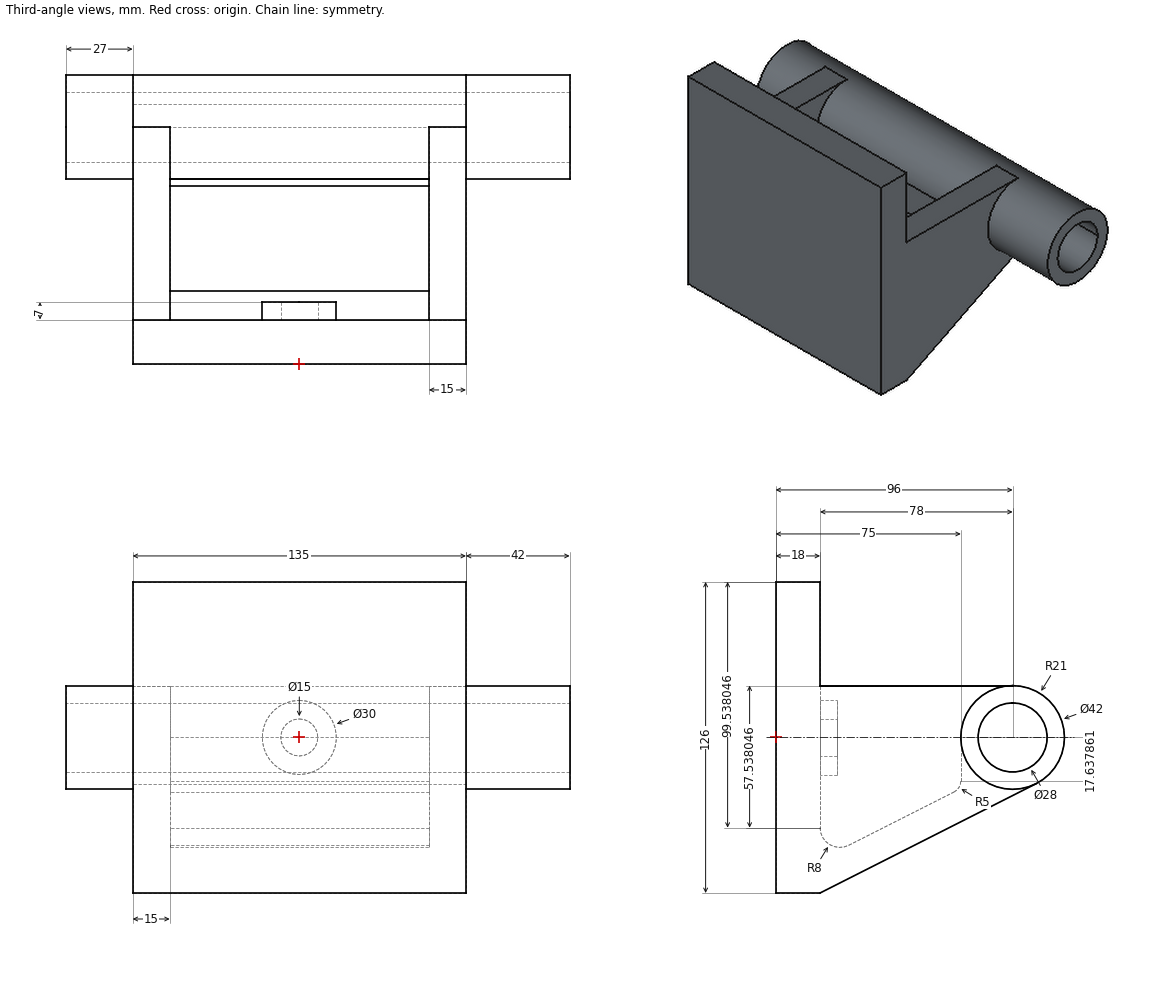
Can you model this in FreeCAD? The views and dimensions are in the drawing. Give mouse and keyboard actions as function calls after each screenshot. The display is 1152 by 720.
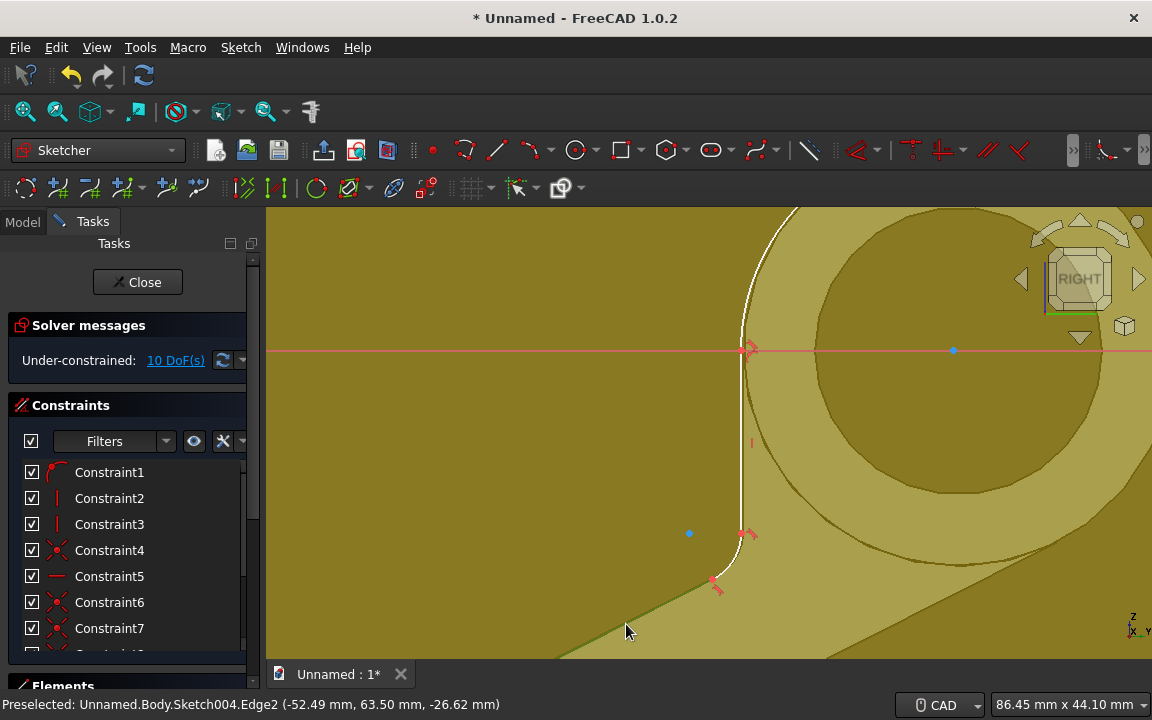
scroll(782, 405, down, 4)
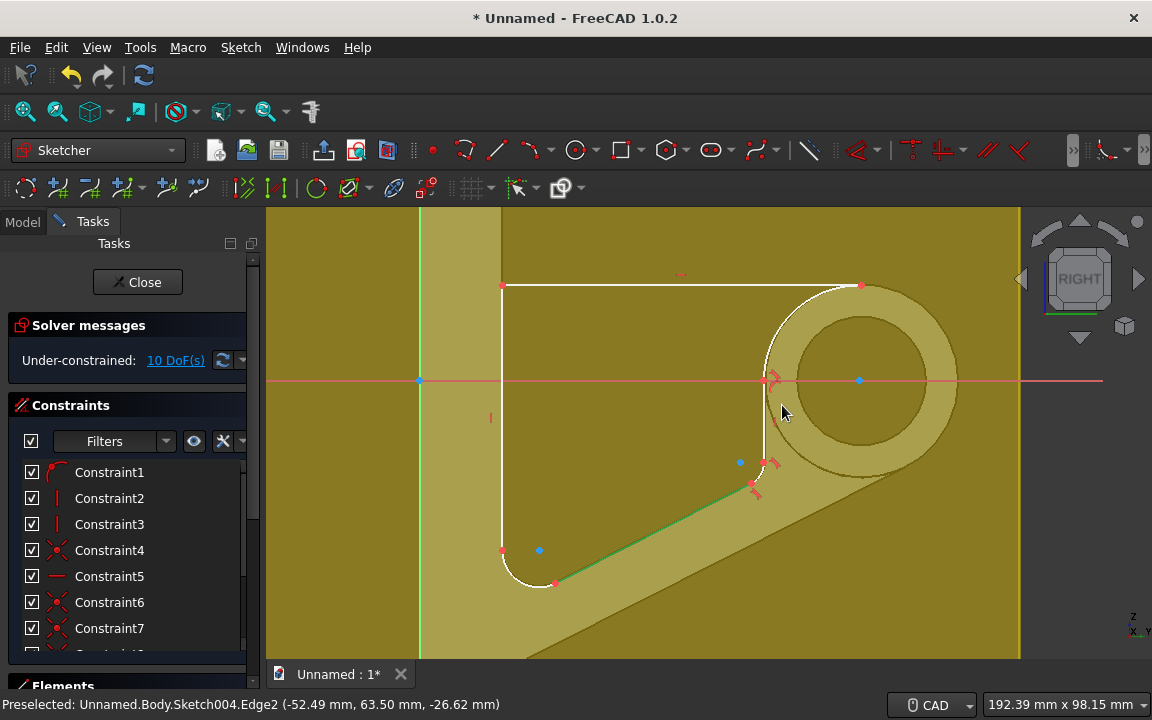
click(509, 571)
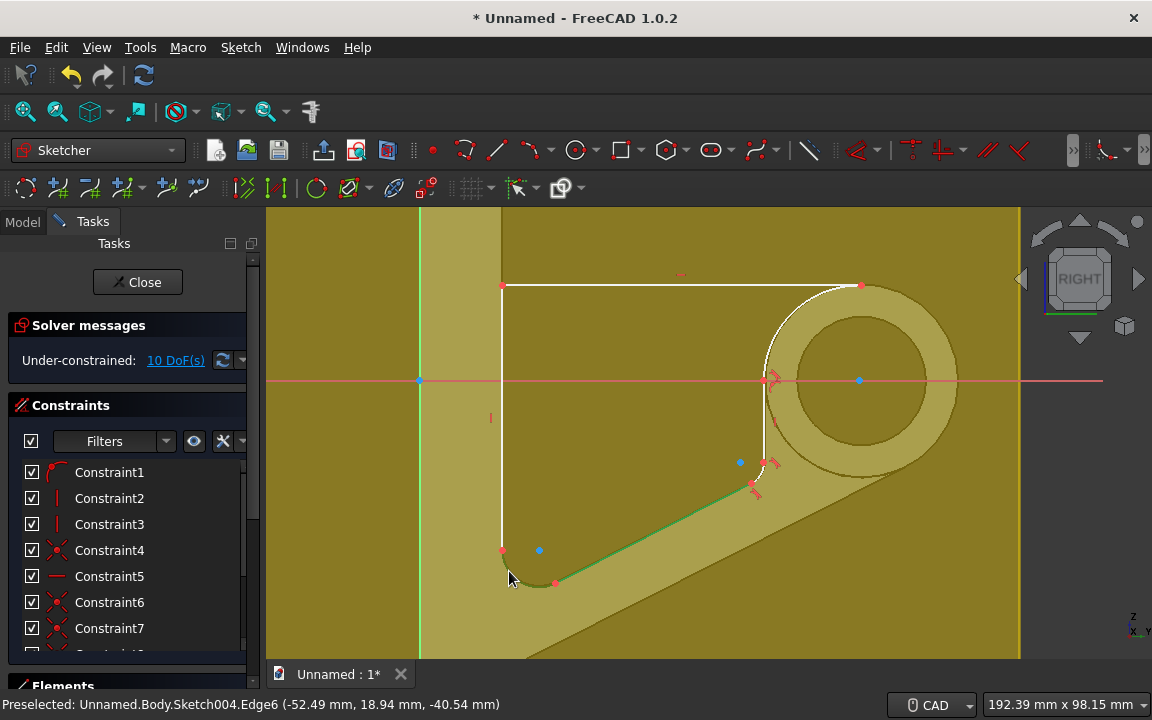
key(t)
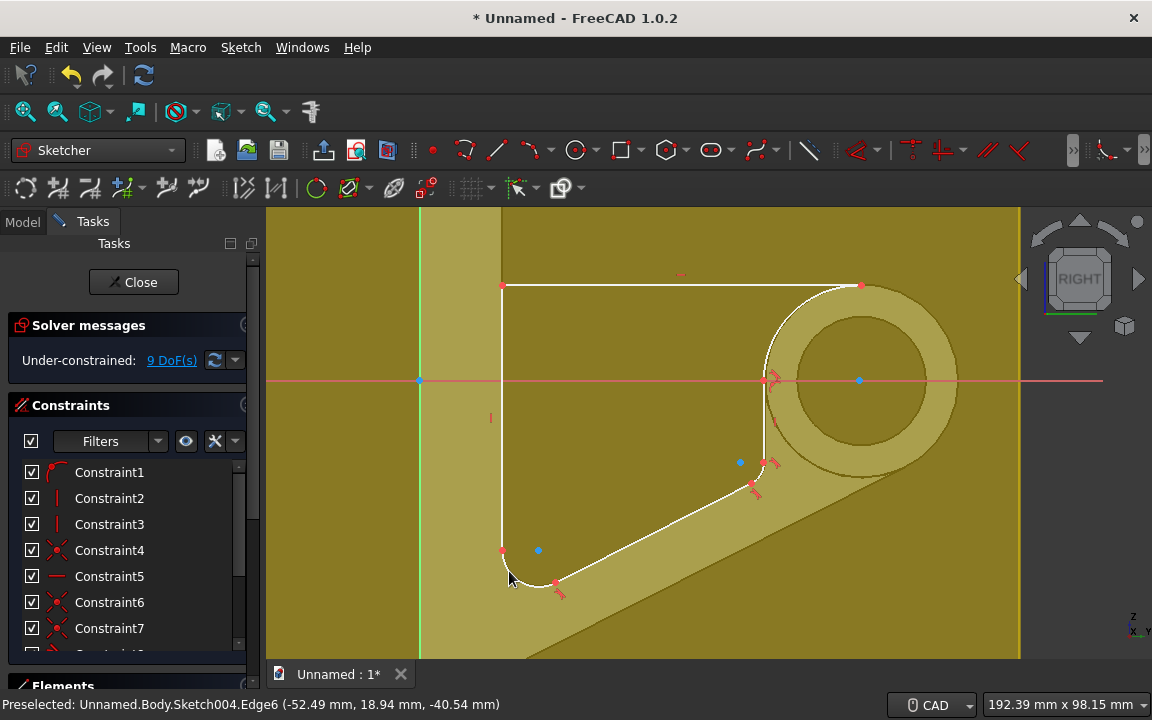
click(502, 471)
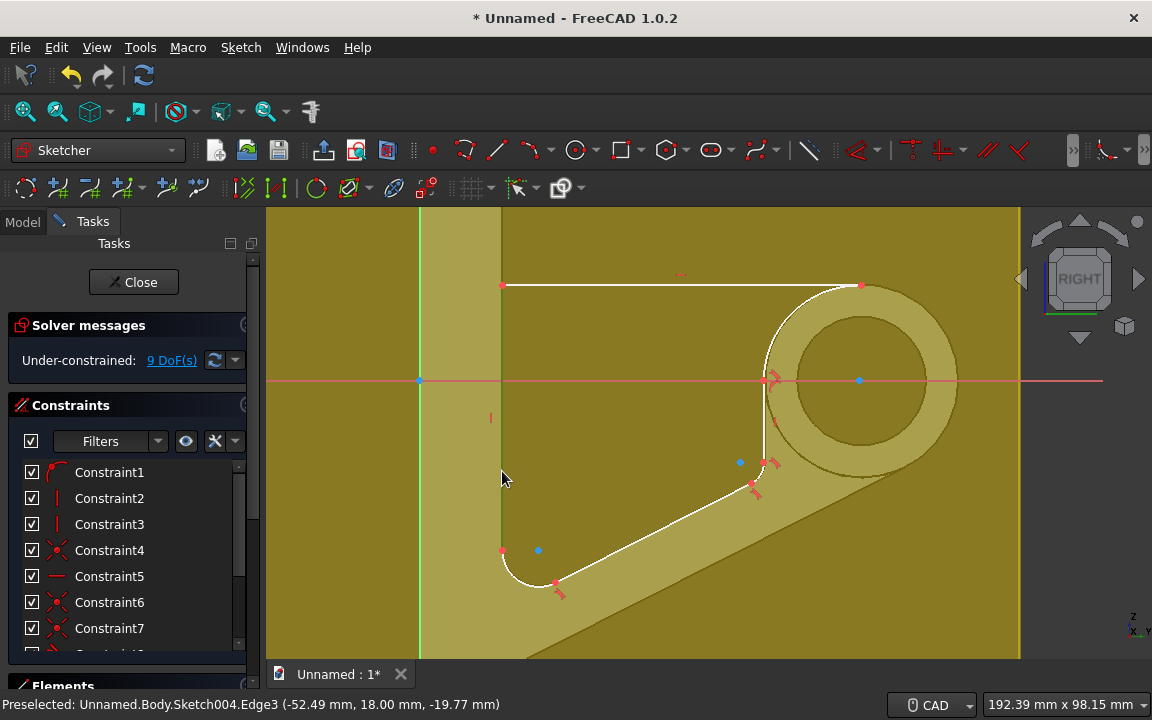
click(509, 571)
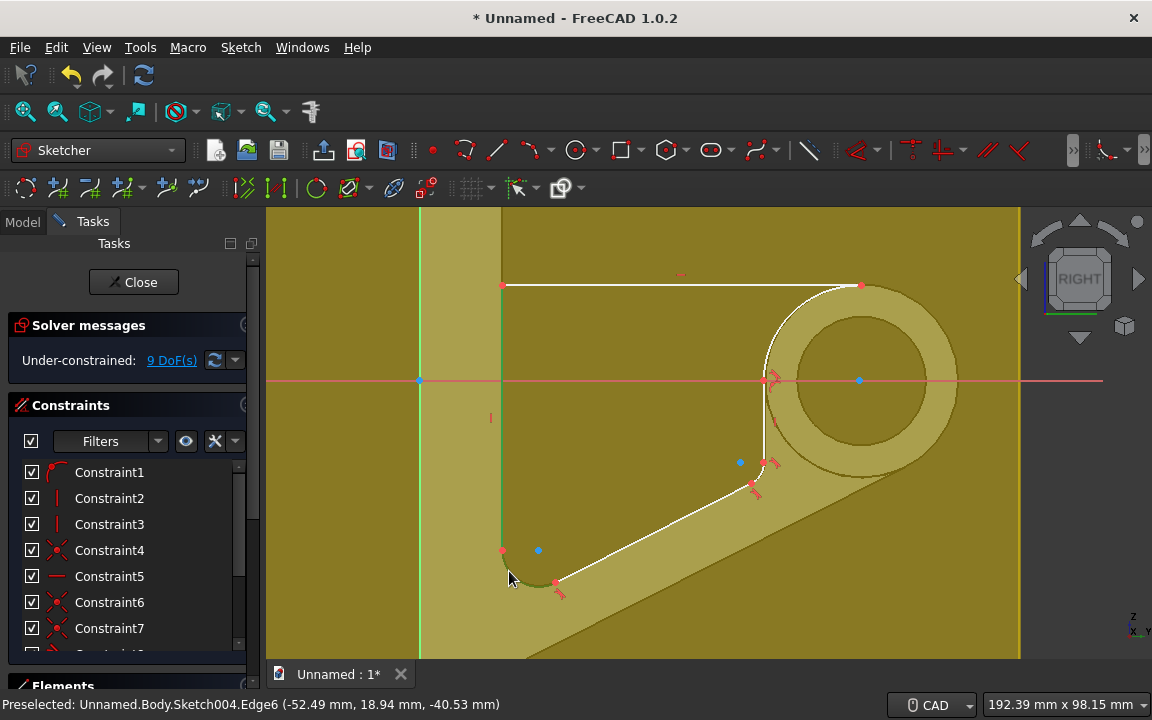
key(t)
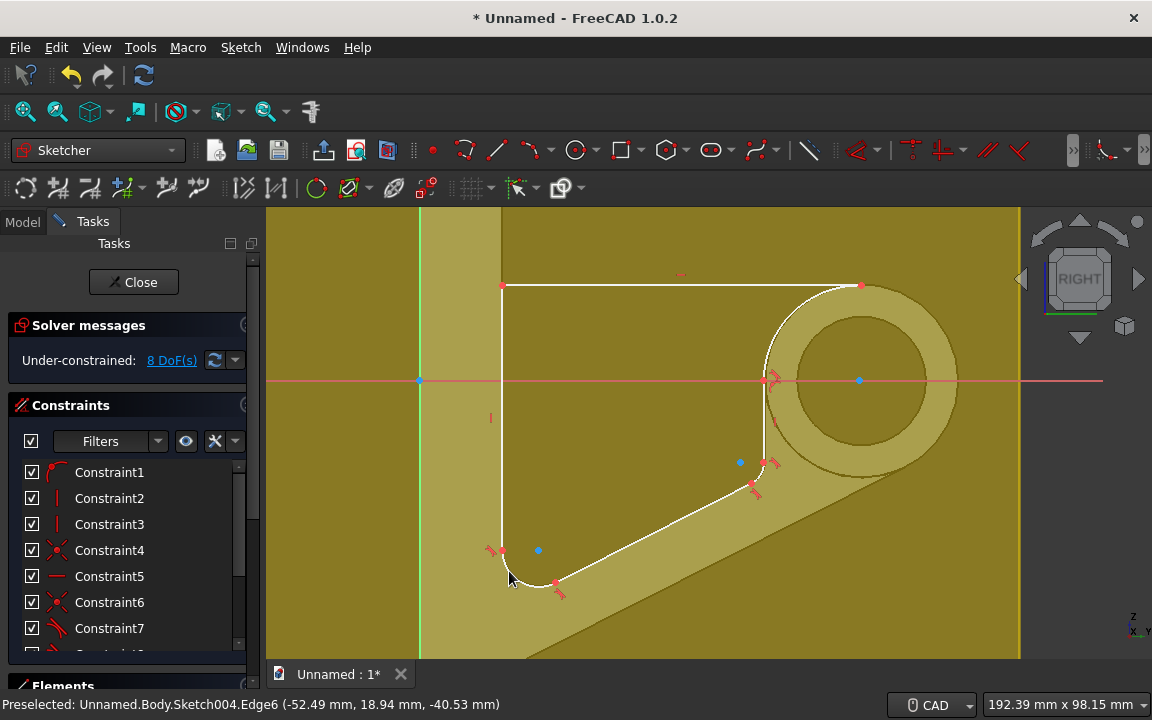
click(610, 285)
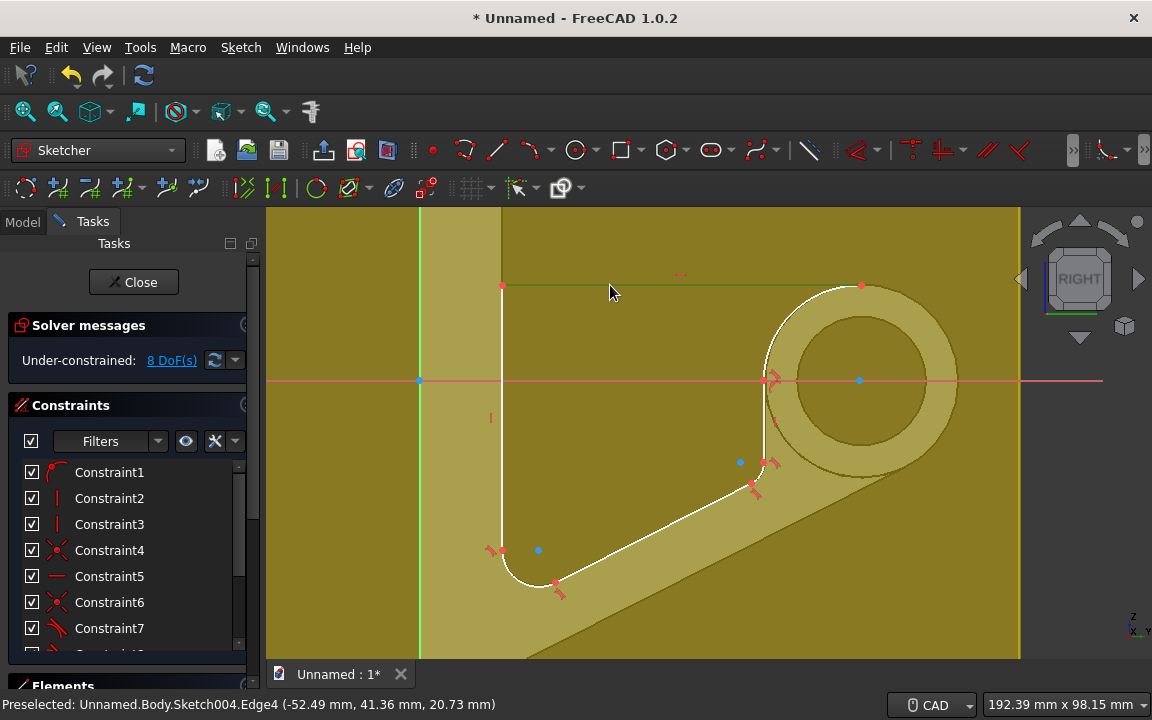
scroll(817, 295, up, 2)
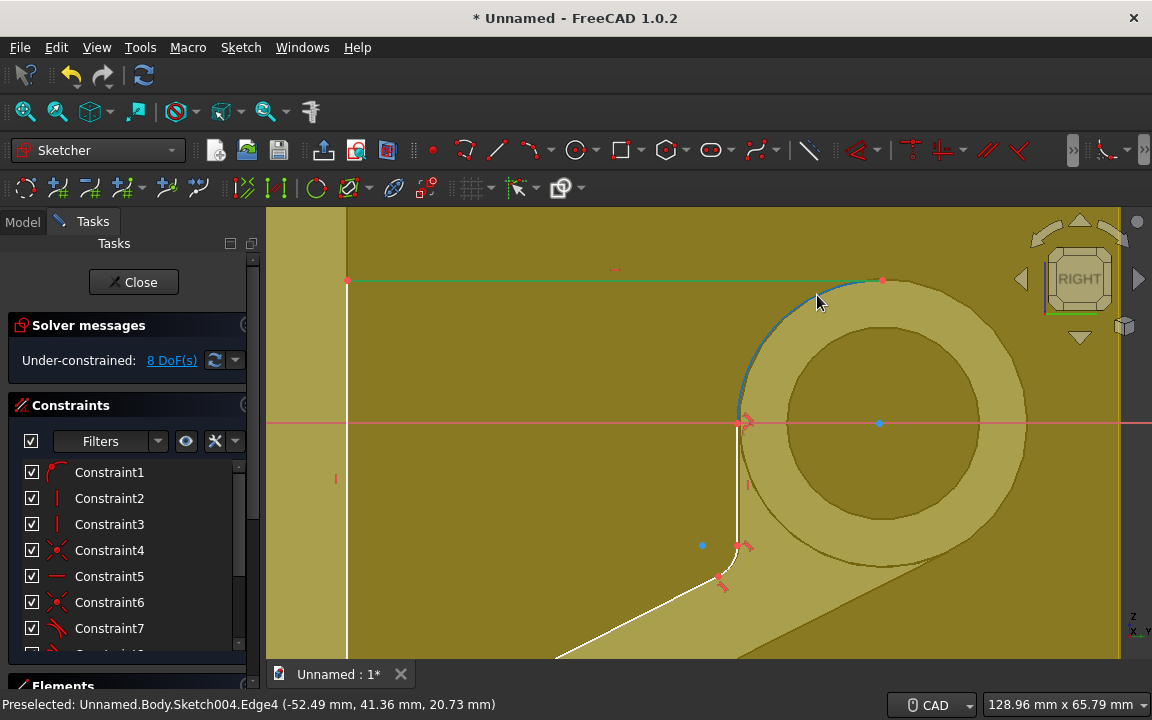
click(817, 295)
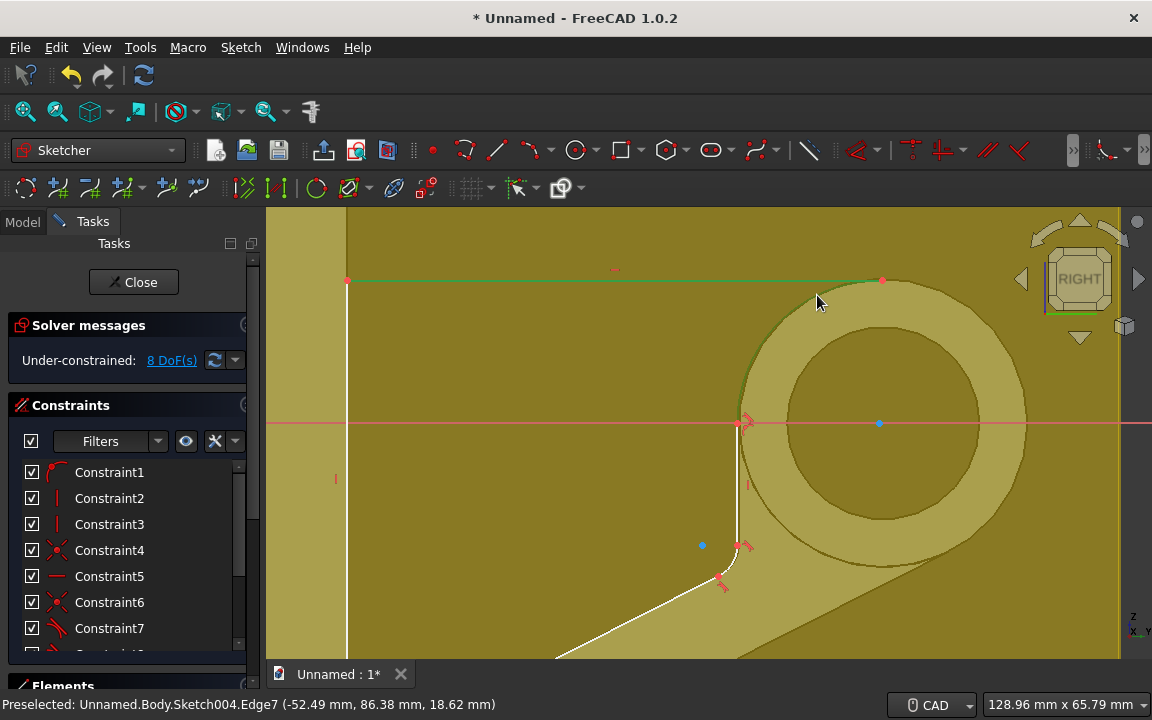
key(t)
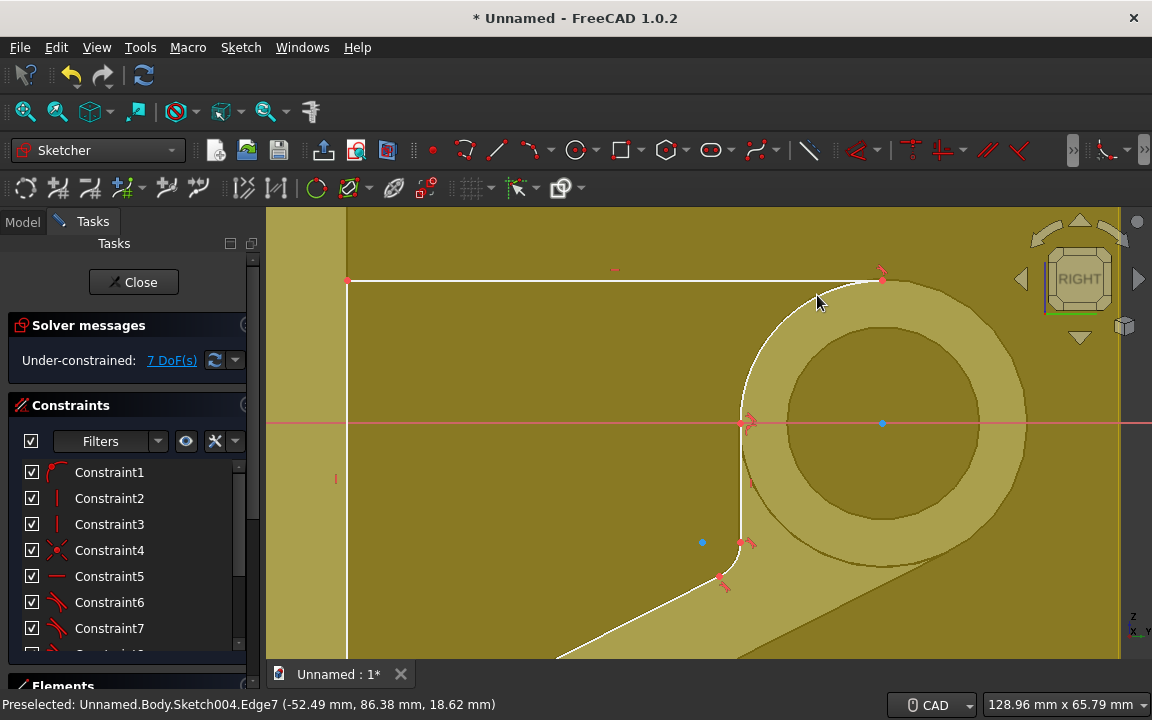
click(856, 150)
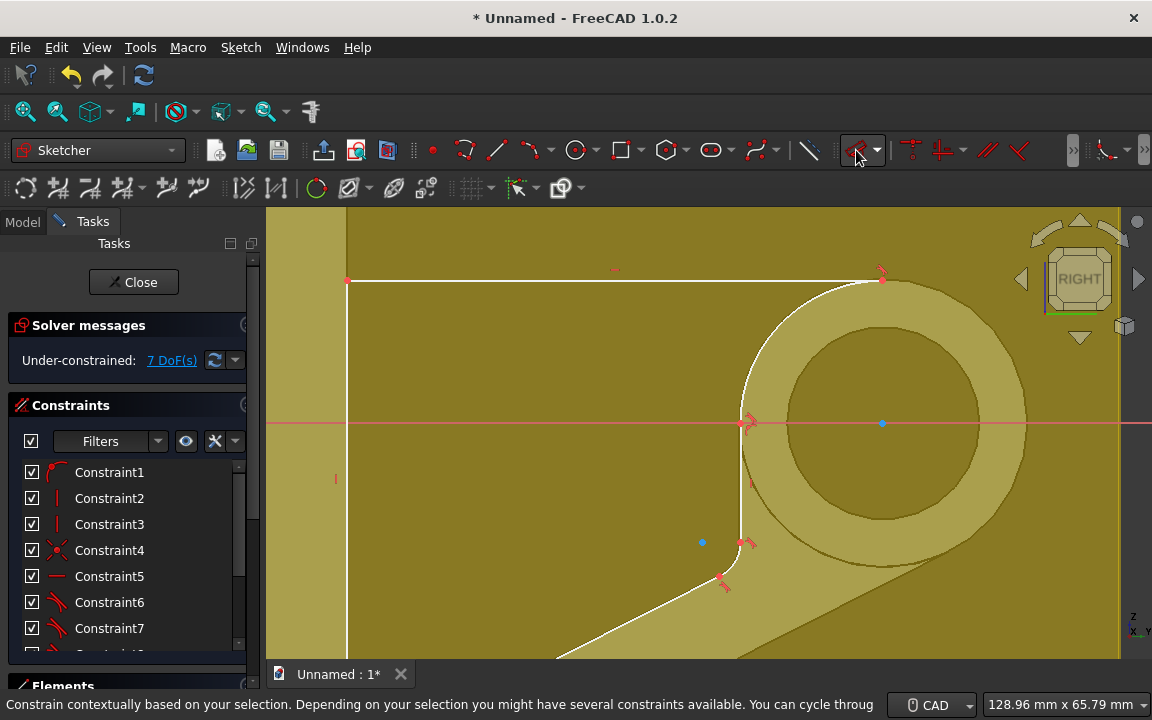
click(730, 569)
click(753, 591)